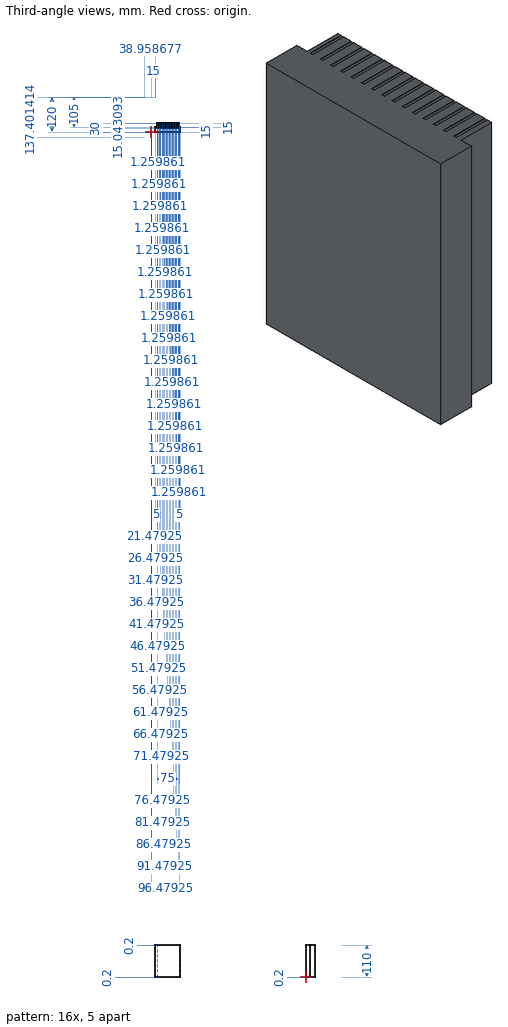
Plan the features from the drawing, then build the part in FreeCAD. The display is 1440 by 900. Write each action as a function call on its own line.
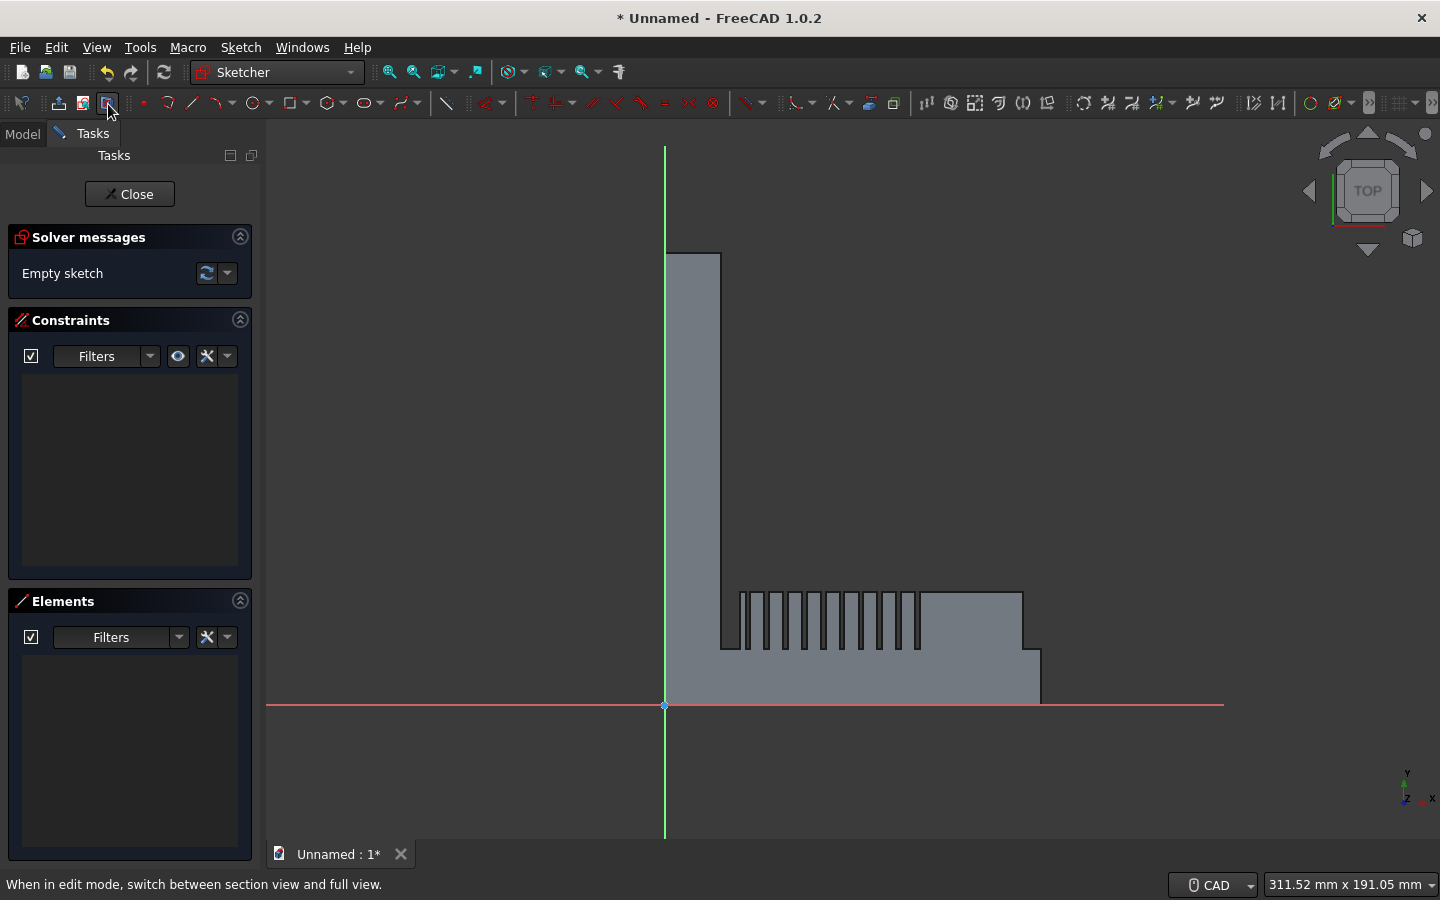
scroll(955, 638, up, 11)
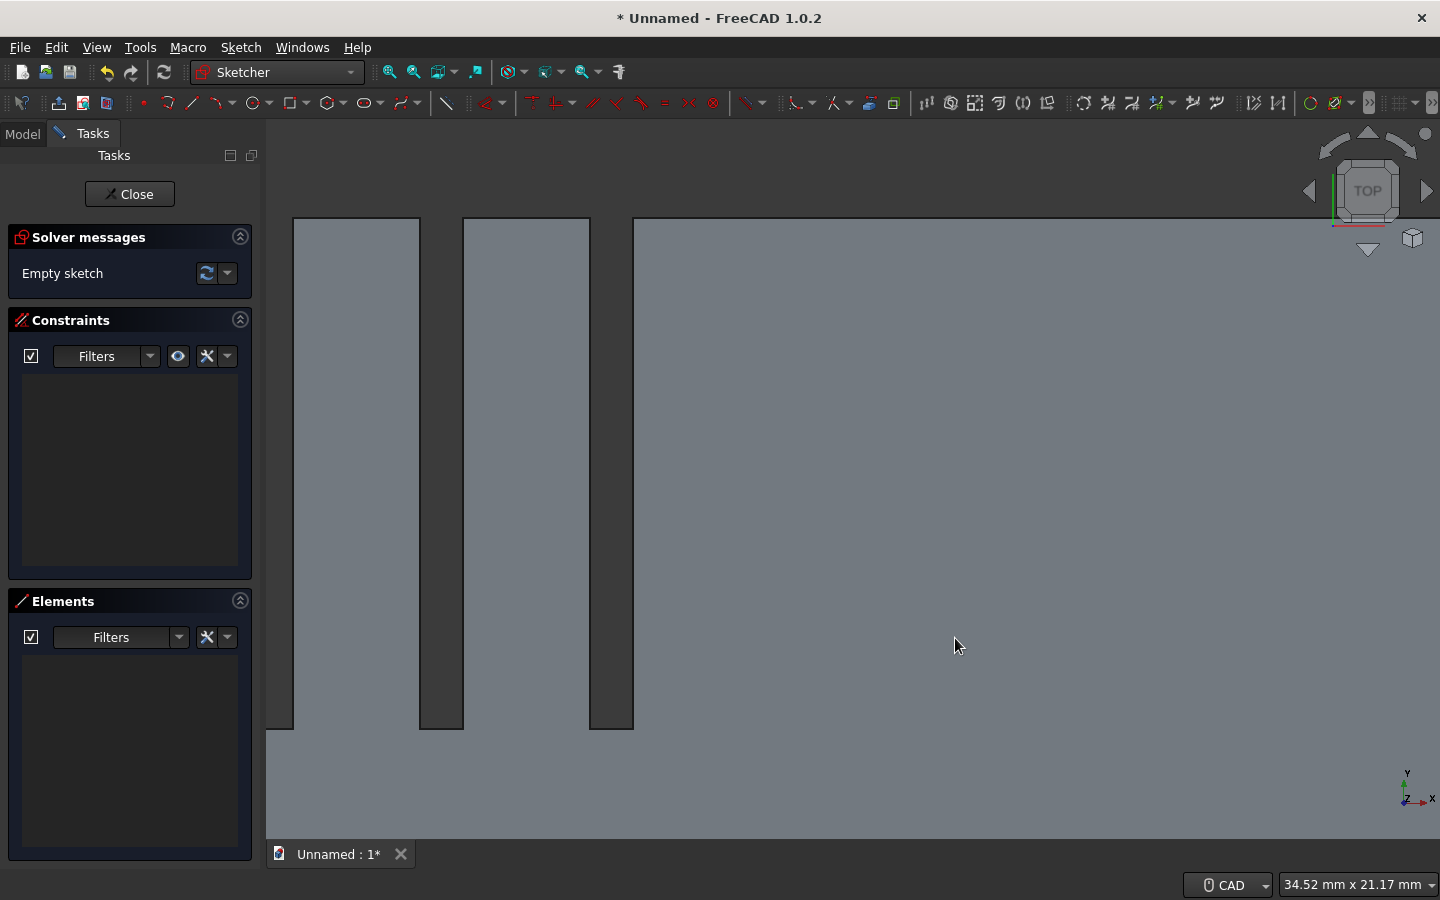
click(290, 104)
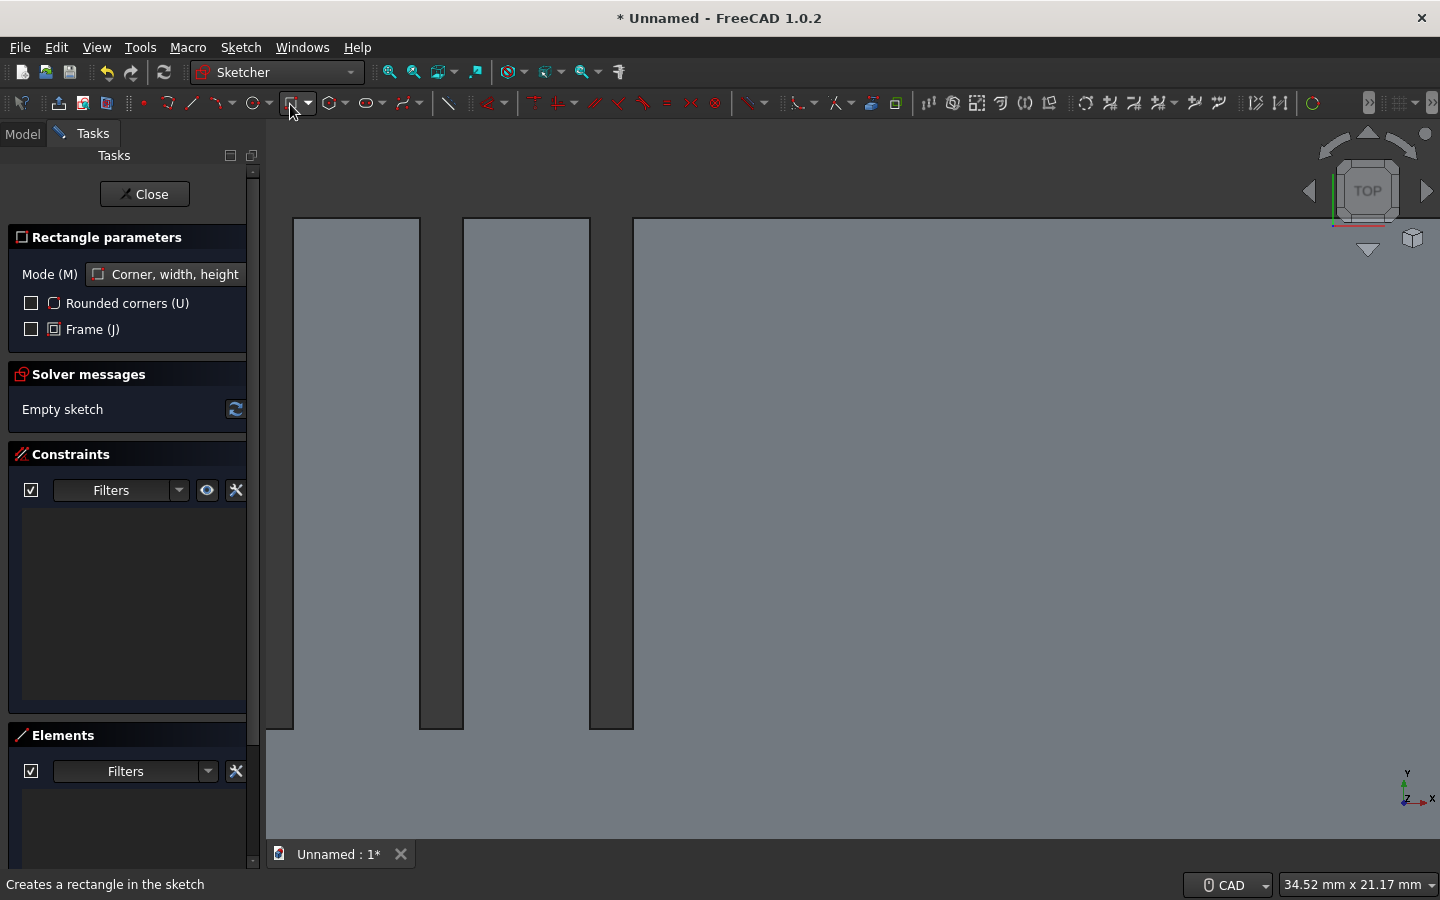
click(760, 218)
click(803, 729)
key(Escape)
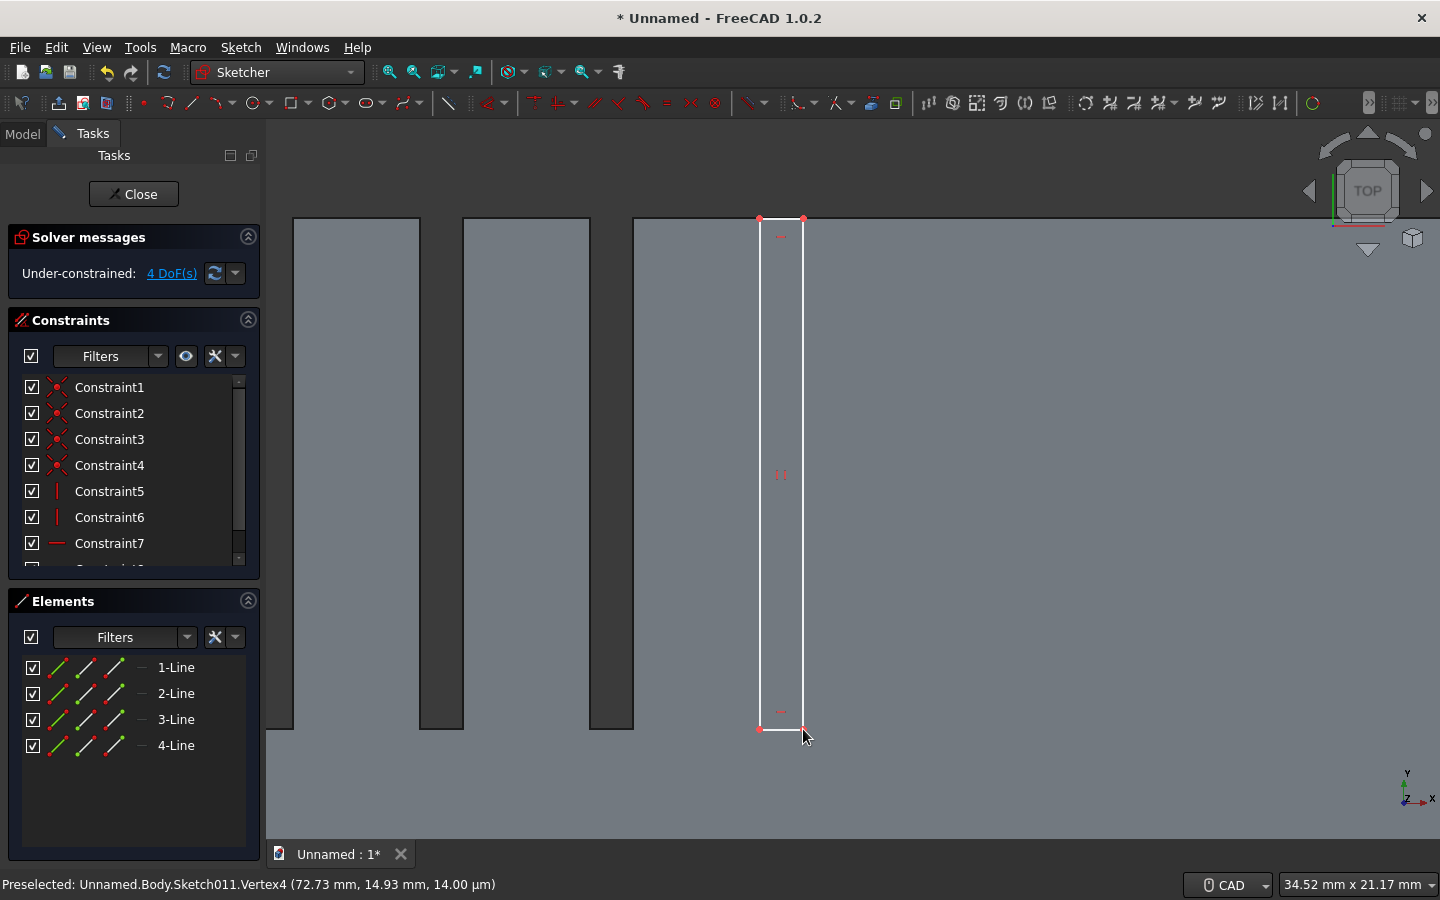
click(488, 104)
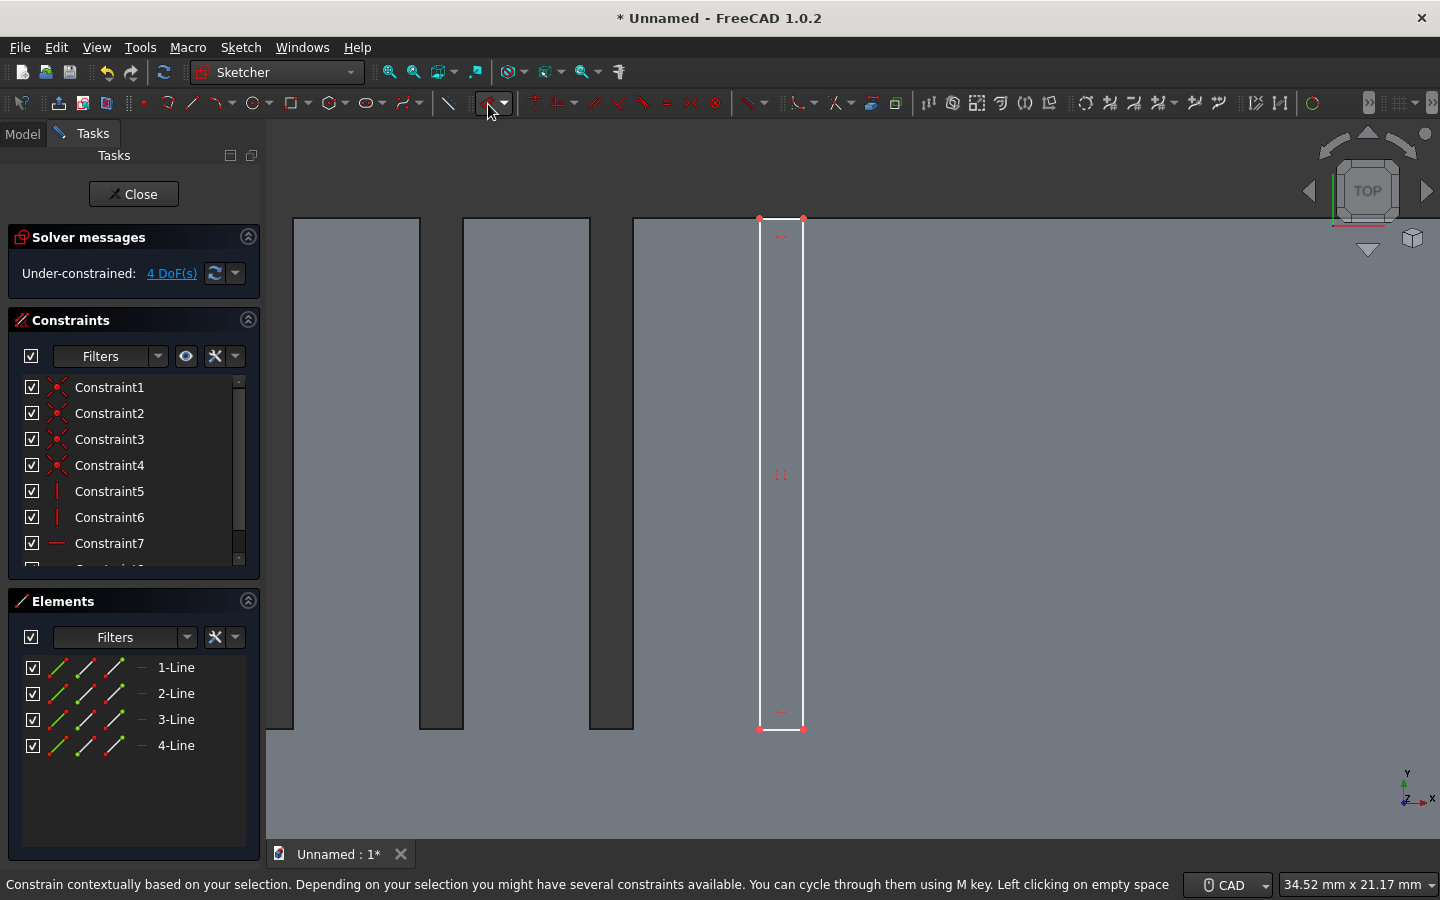
click(760, 219)
click(818, 515)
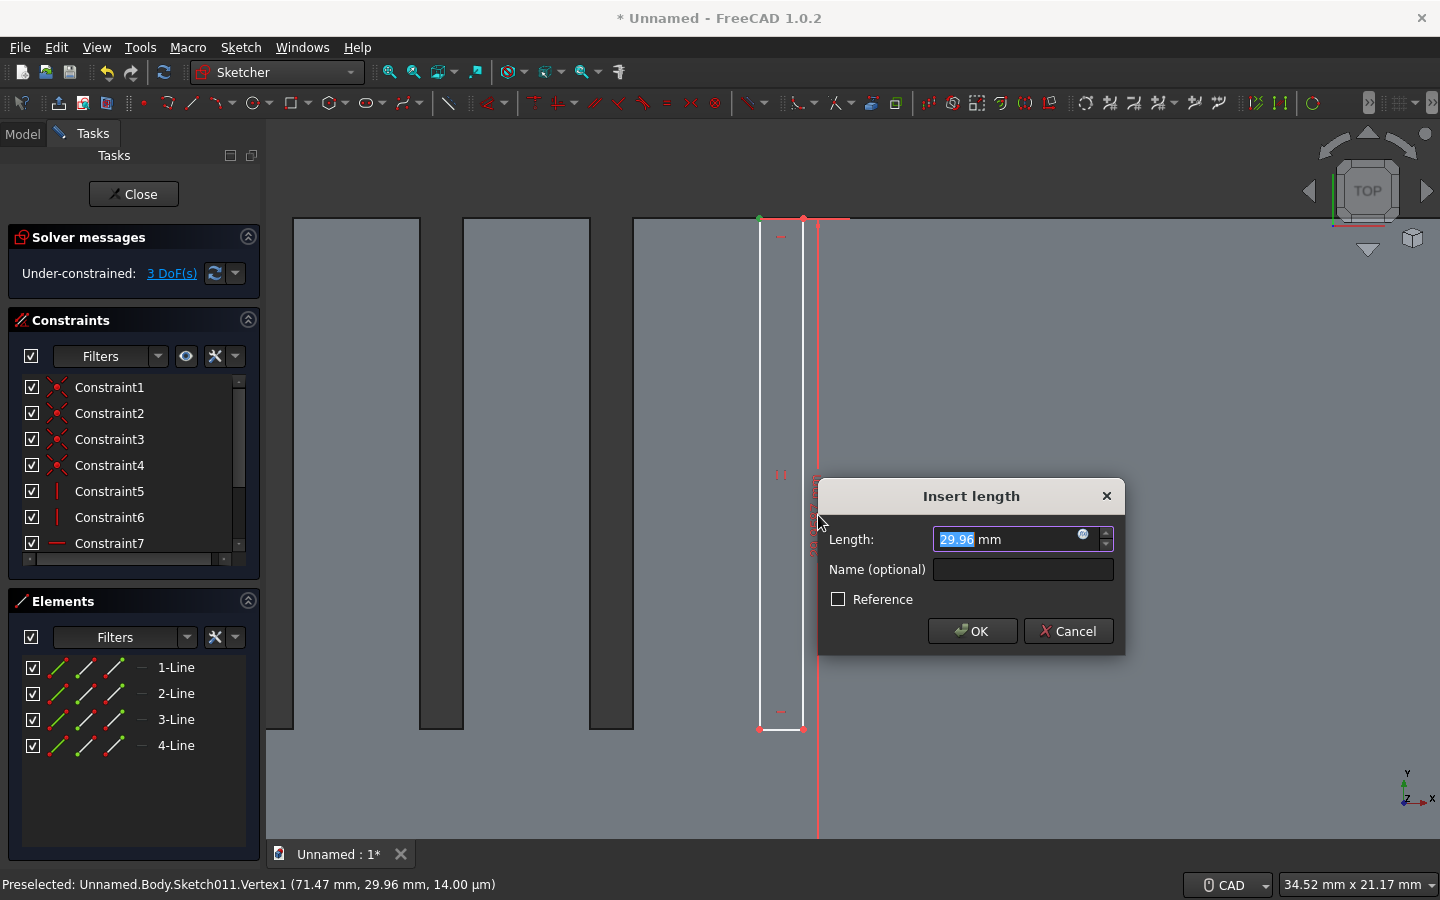
text(30)
key(Return)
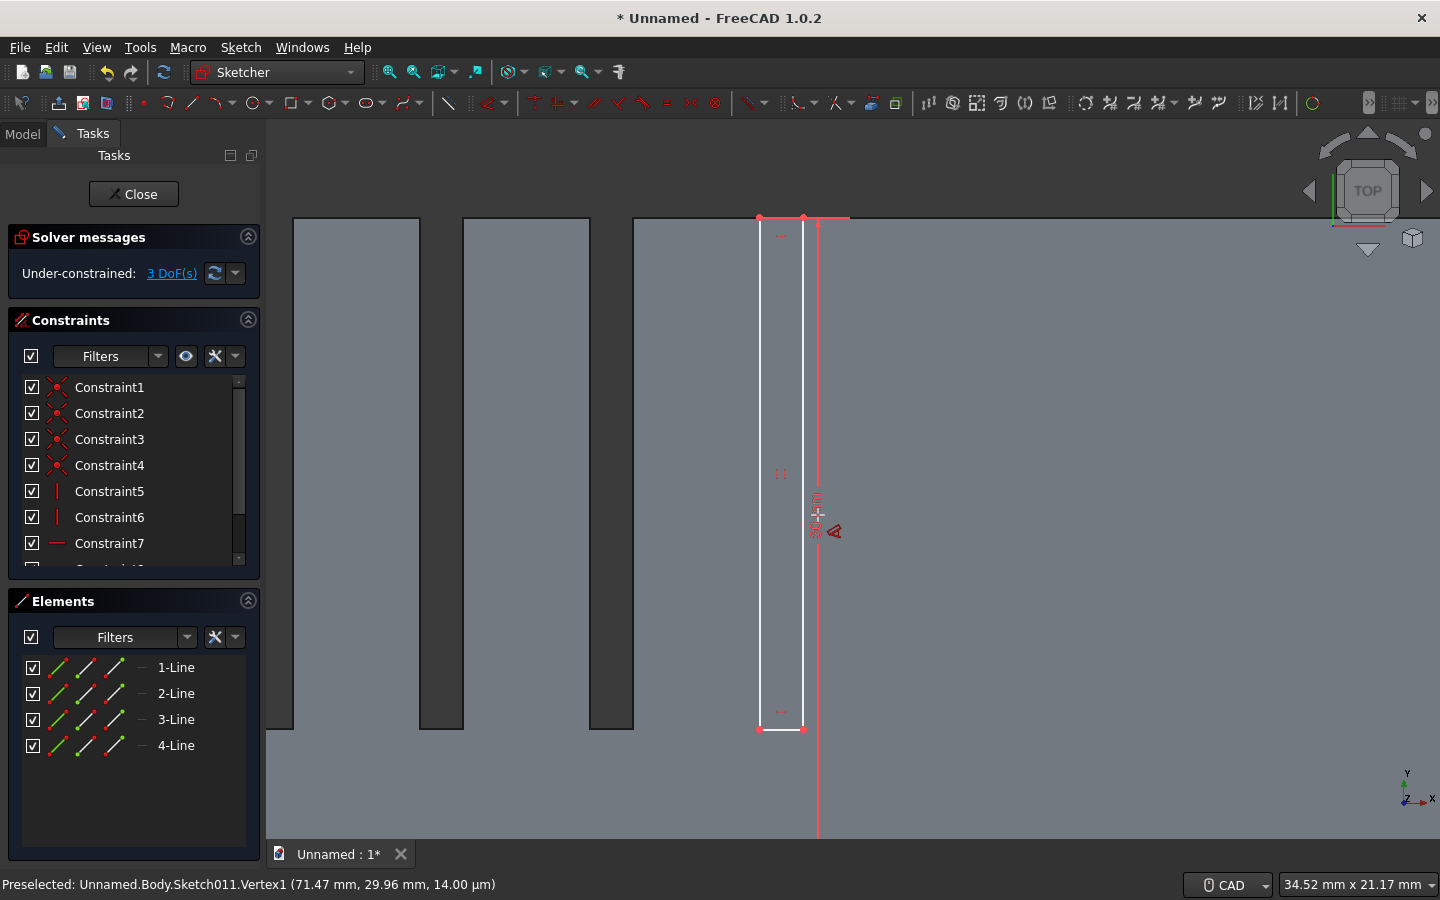
click(773, 730)
click(781, 764)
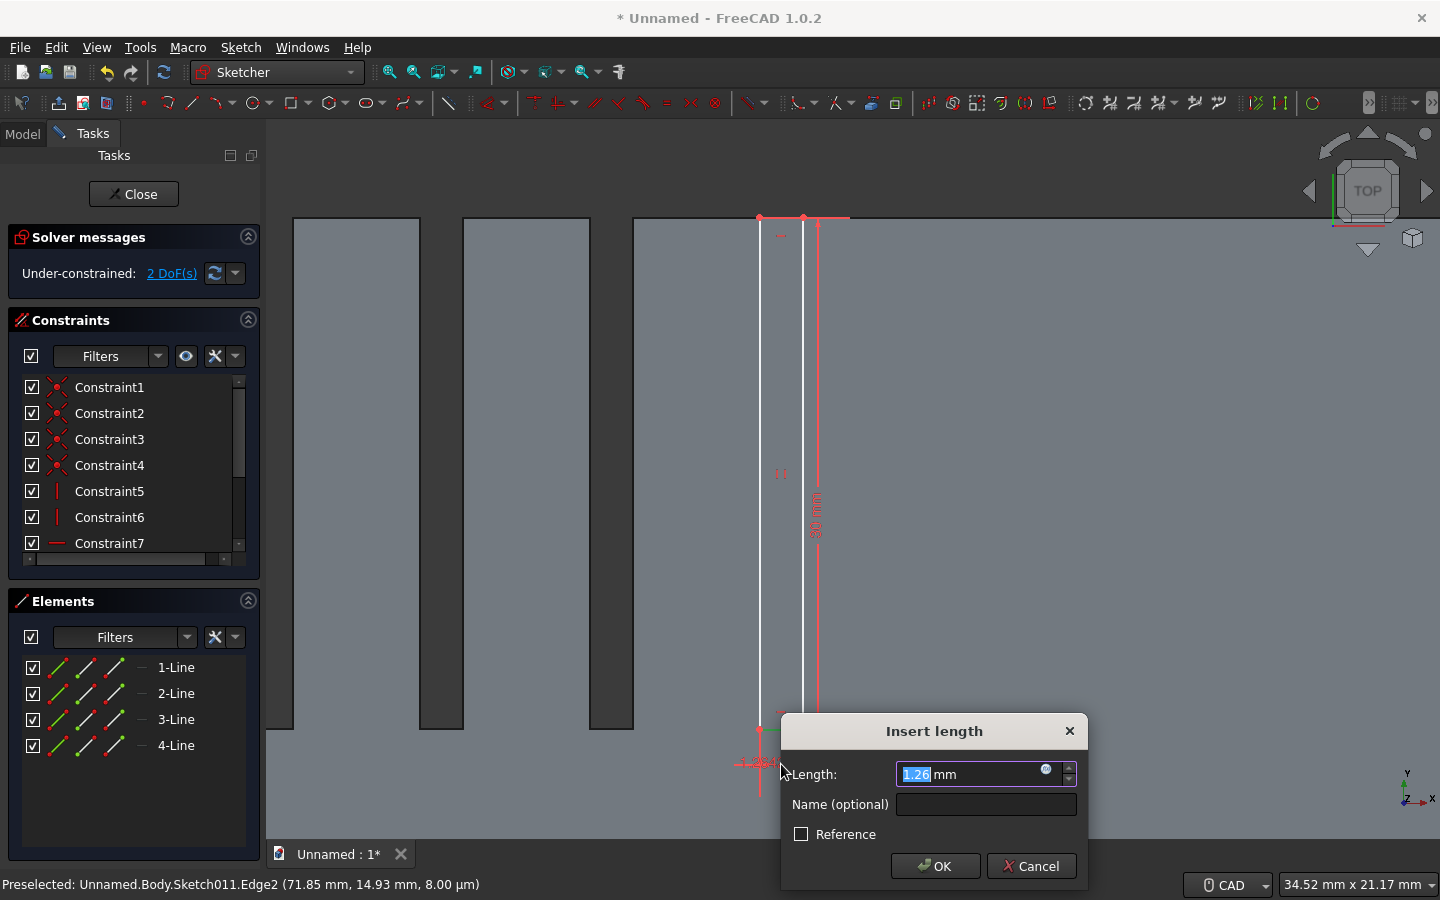
text(1.259861)
key(Return)